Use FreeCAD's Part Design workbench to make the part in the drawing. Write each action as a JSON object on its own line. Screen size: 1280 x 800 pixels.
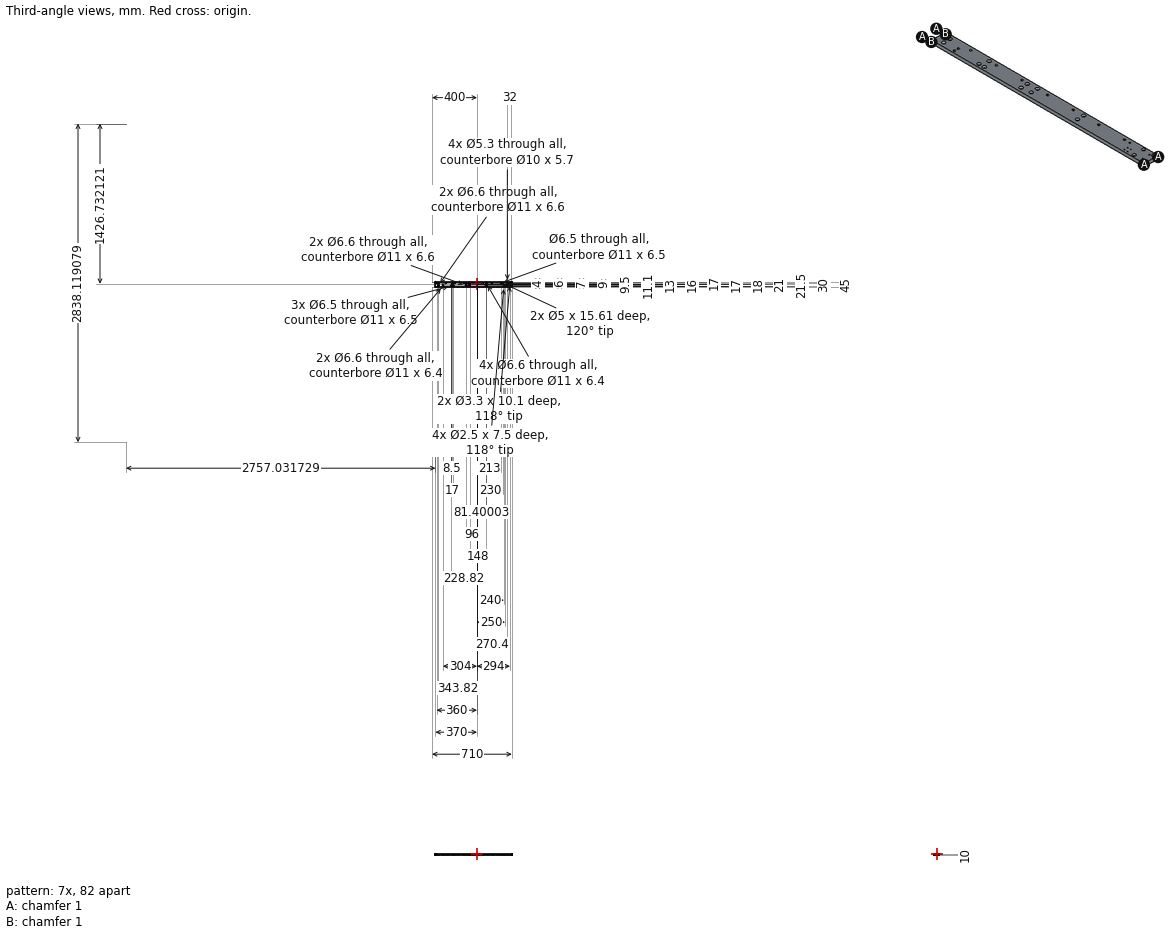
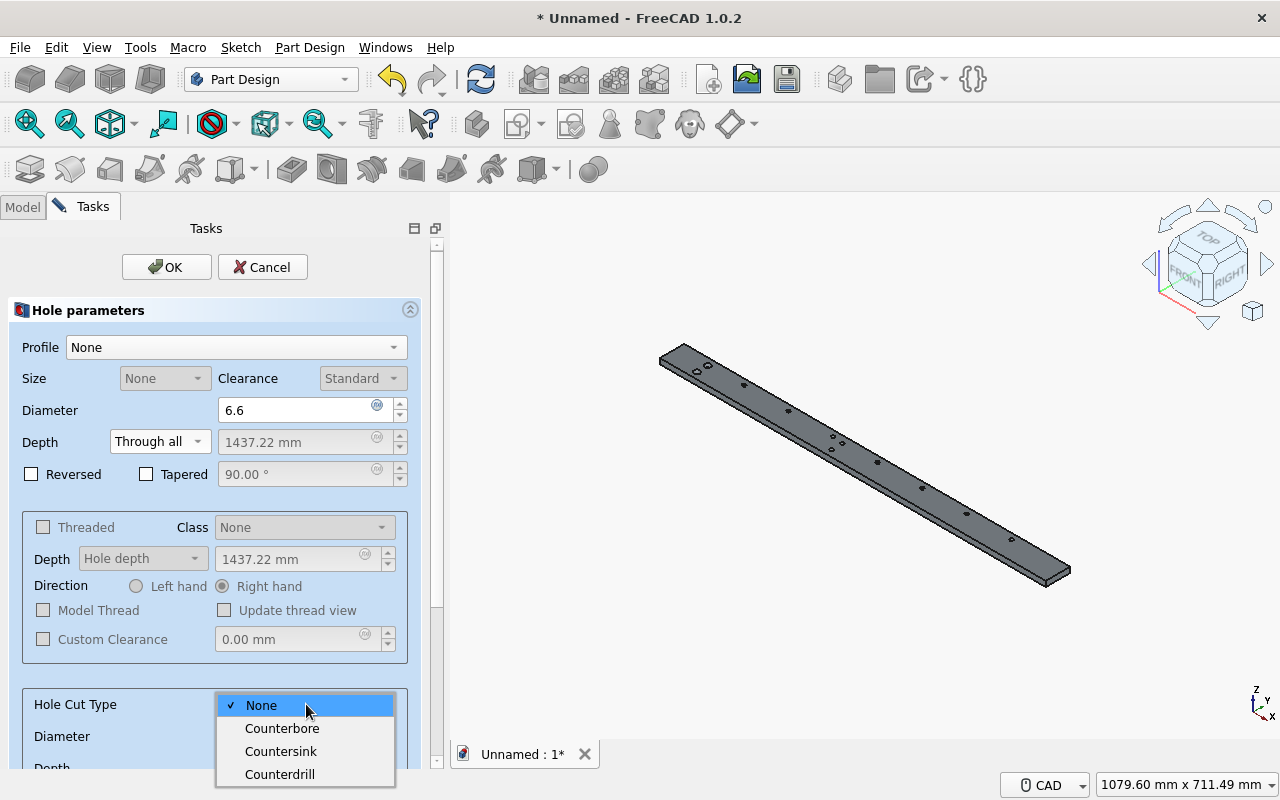
{"action": "left_click", "coordinate": [304, 728]}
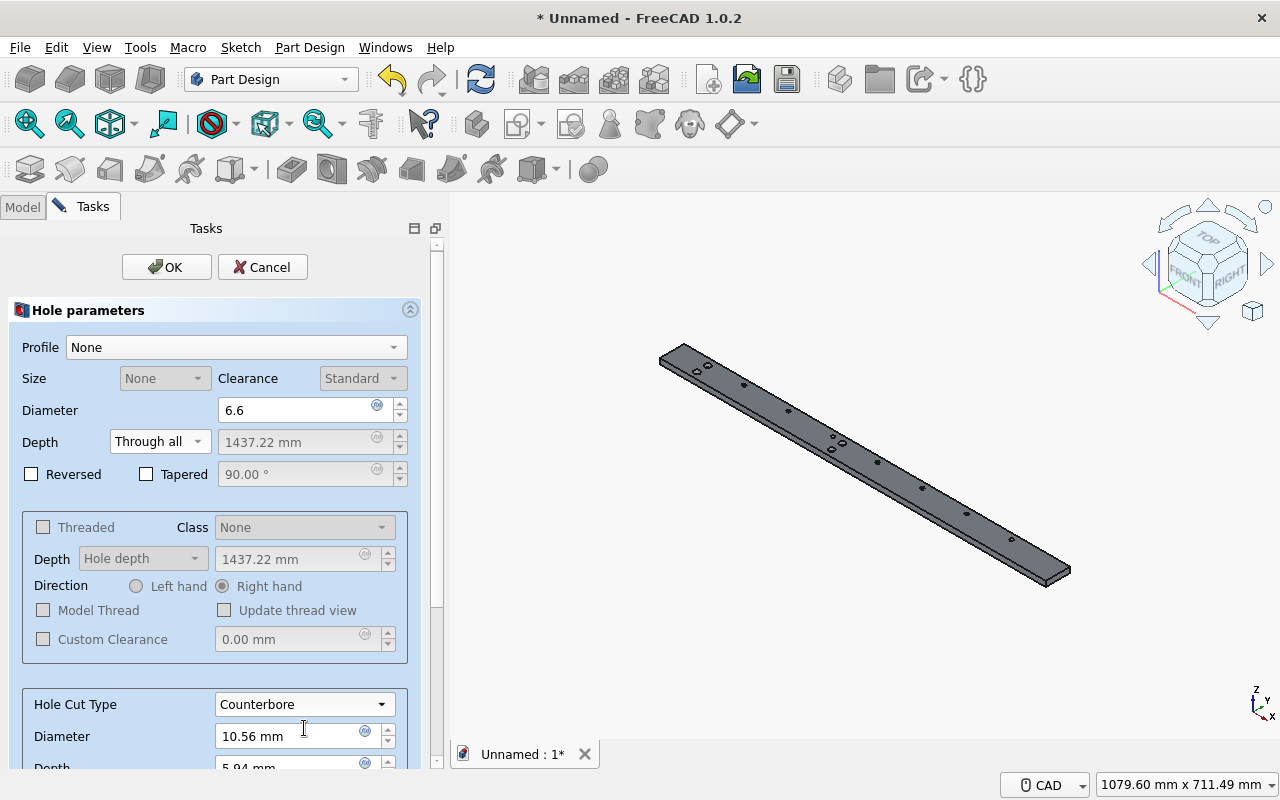
{"action": "triple_click", "coordinate": [298, 736]}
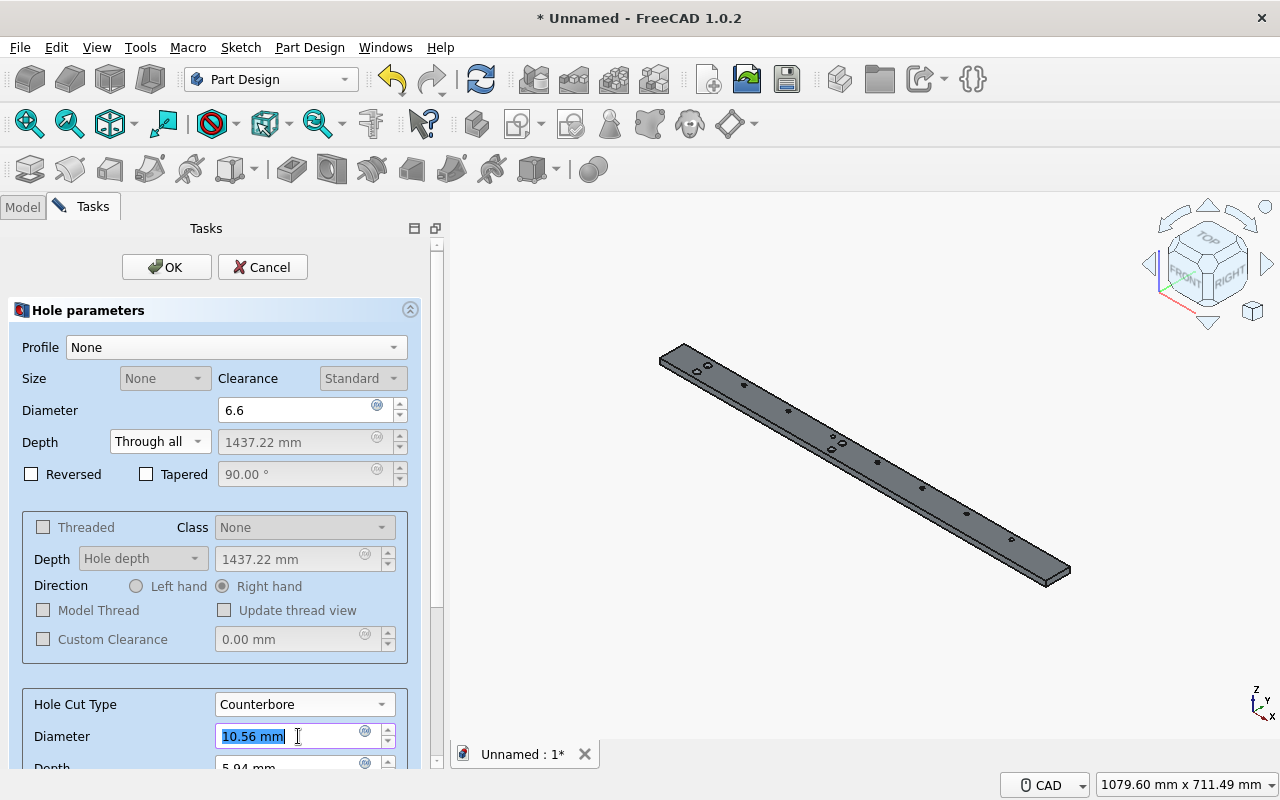
{"action": "type", "text": "11"}
{"action": "key", "text": "Tab"}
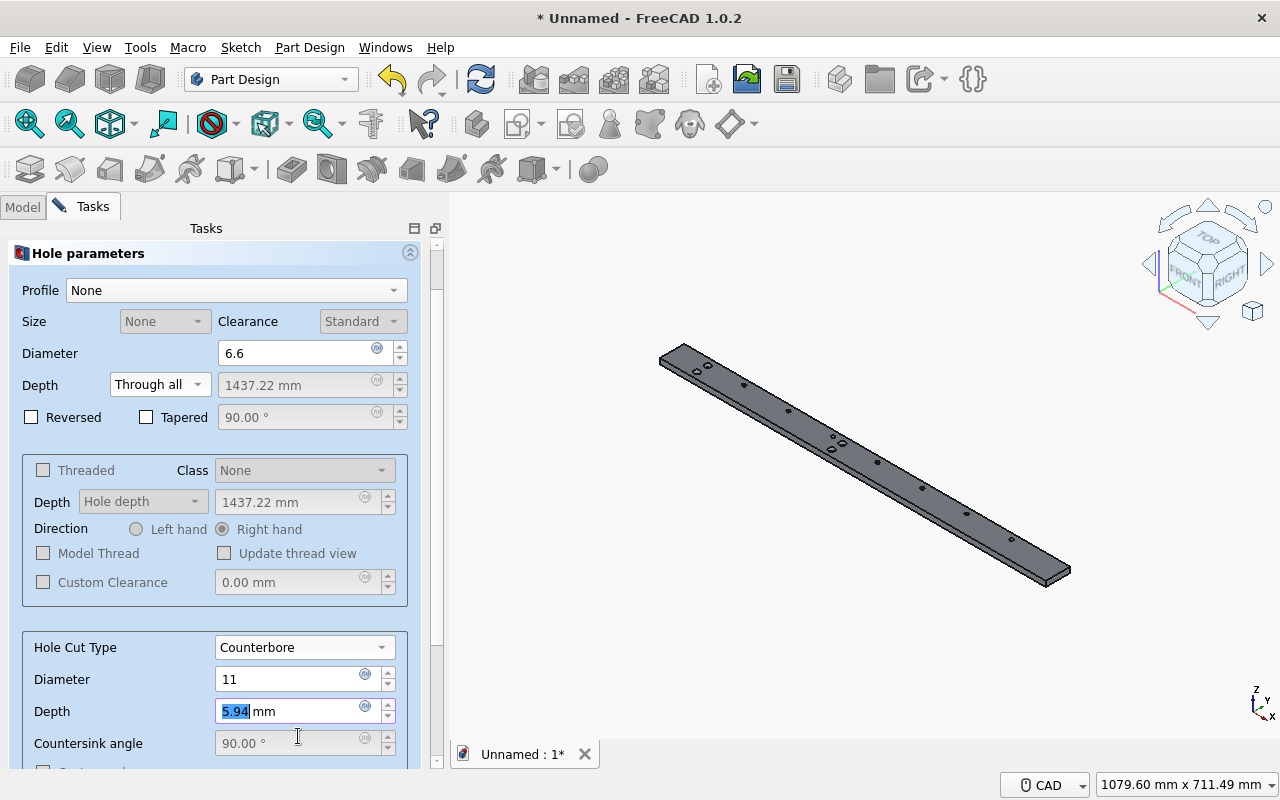
{"action": "type", "text": "6.6"}
{"action": "key", "text": "Tab"}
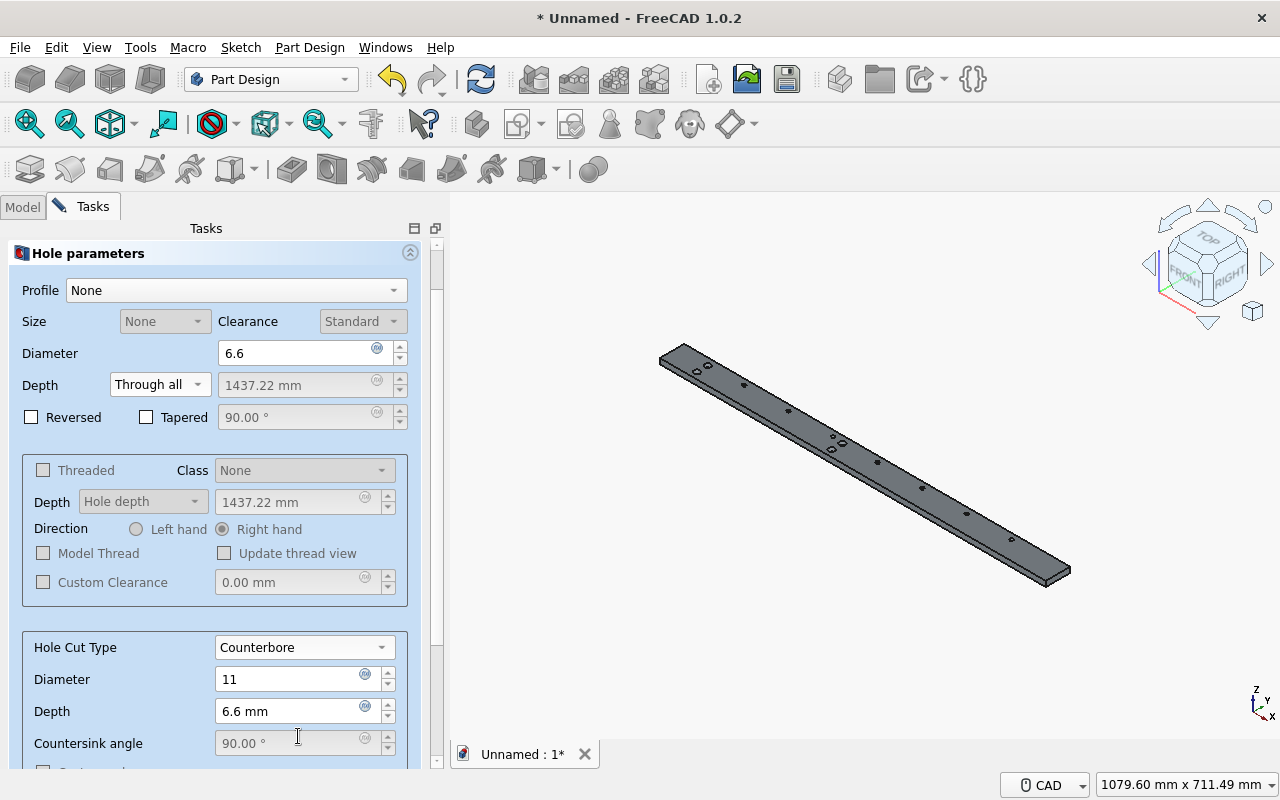
{"action": "scroll", "coordinate": [437, 503], "scroll_direction": "up", "scroll_amount": 2}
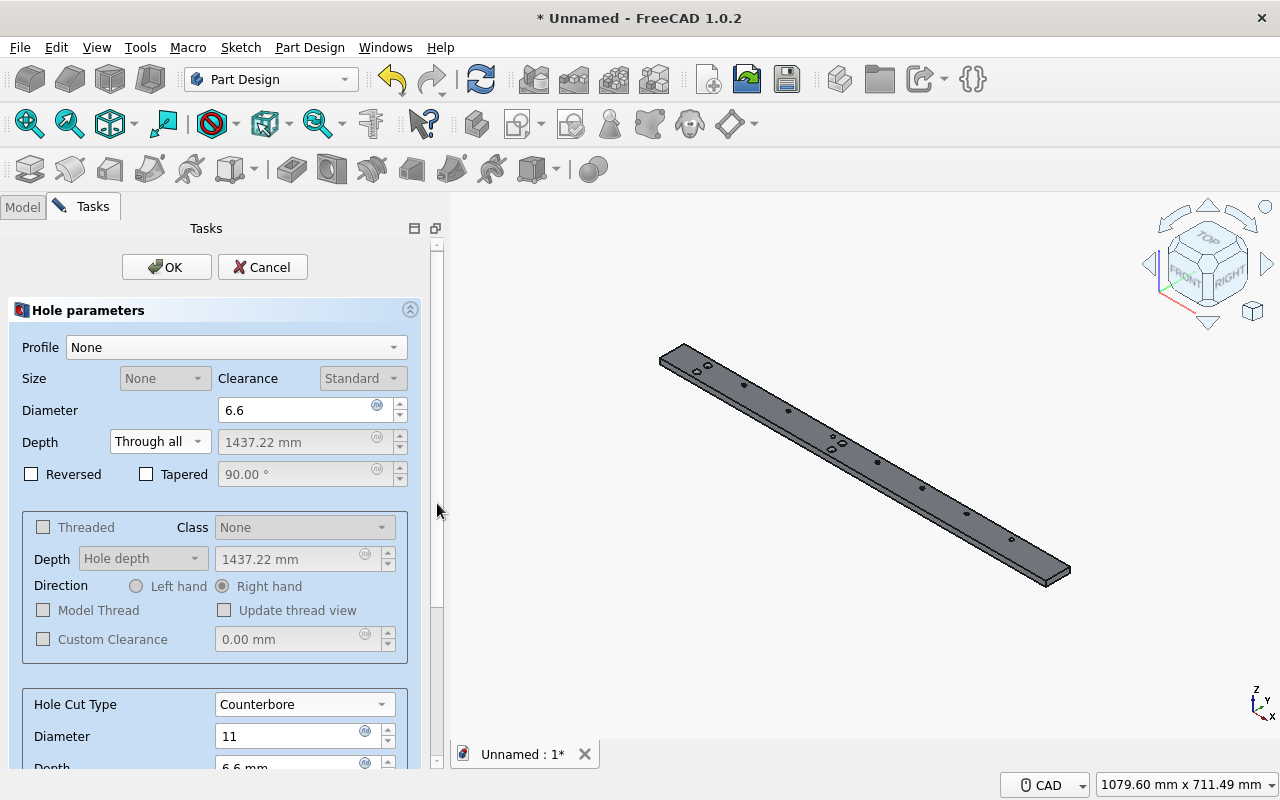
{"action": "left_click", "coordinate": [167, 267]}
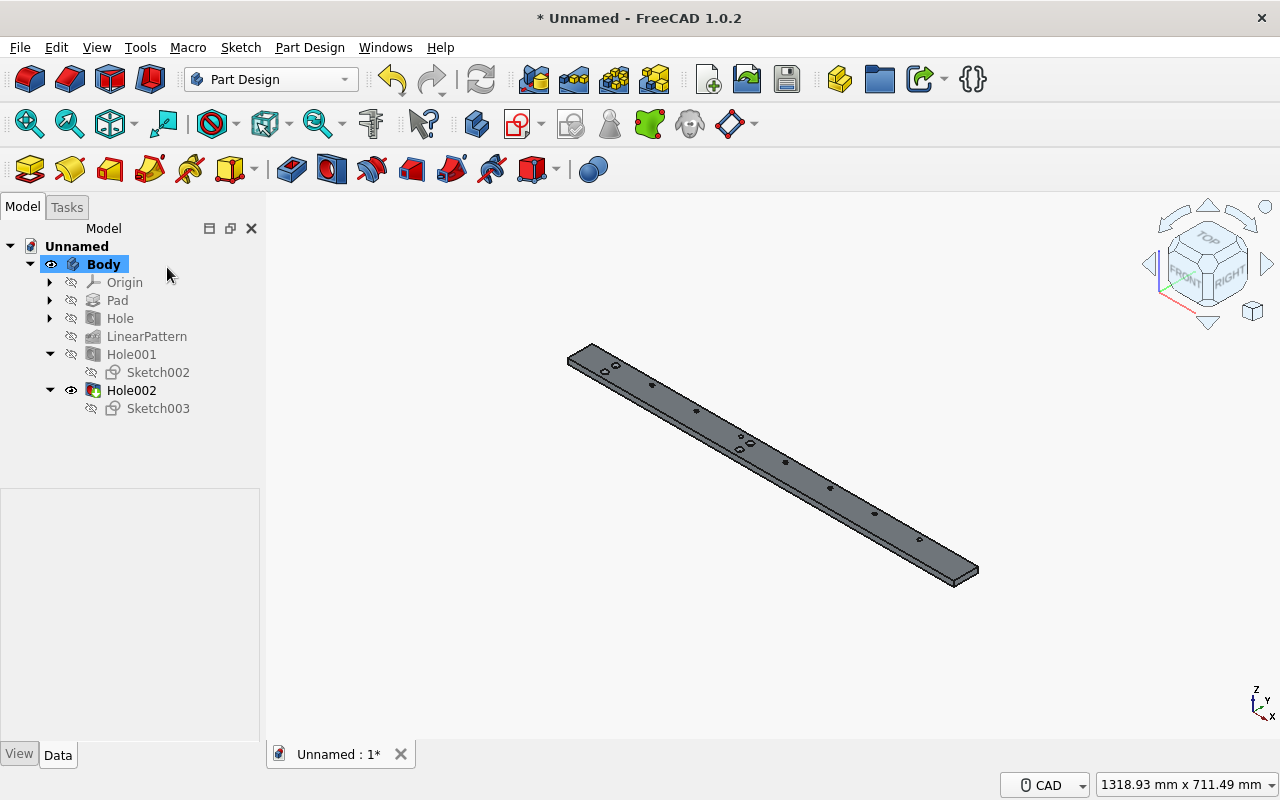
{"action": "left_click", "coordinate": [30, 124]}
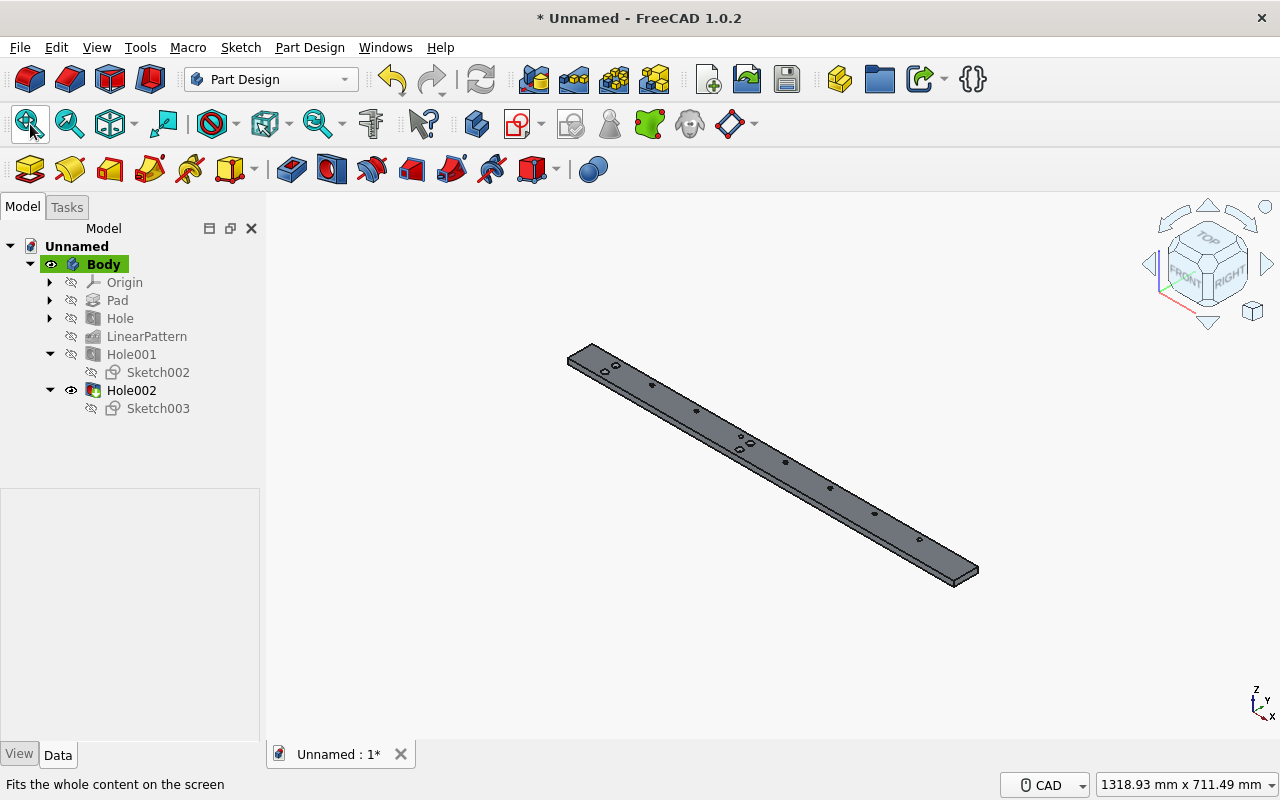
{"action": "left_click", "coordinate": [938, 557]}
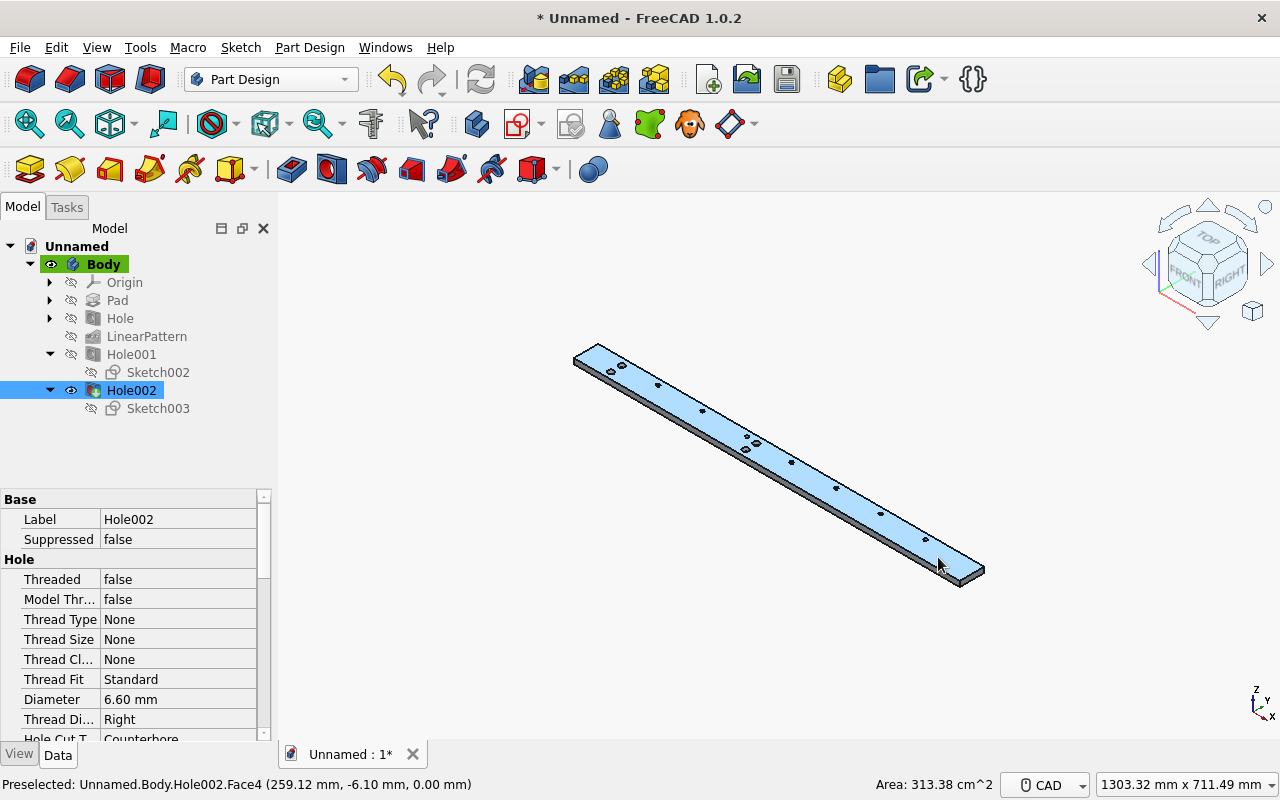
{"action": "left_click", "coordinate": [518, 124]}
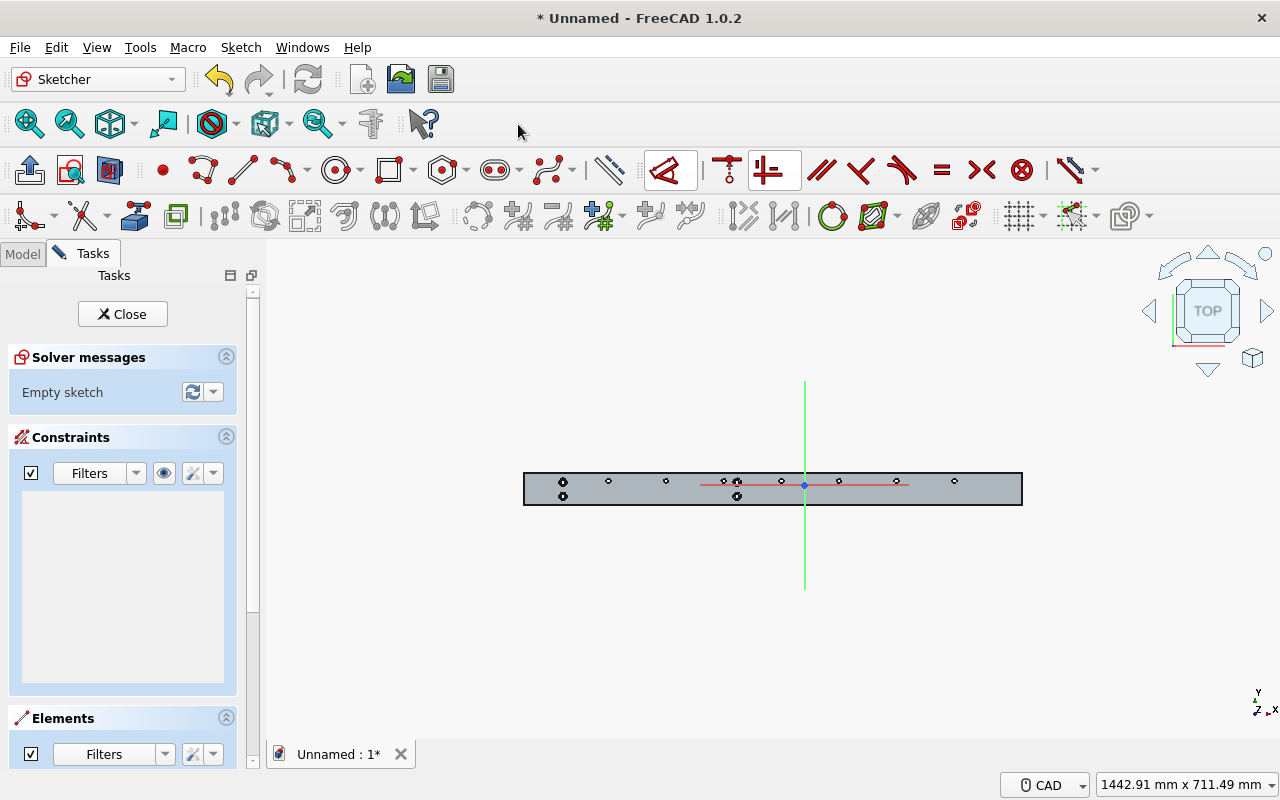
{"action": "scroll", "coordinate": [645, 489], "scroll_direction": "up", "scroll_amount": 13}